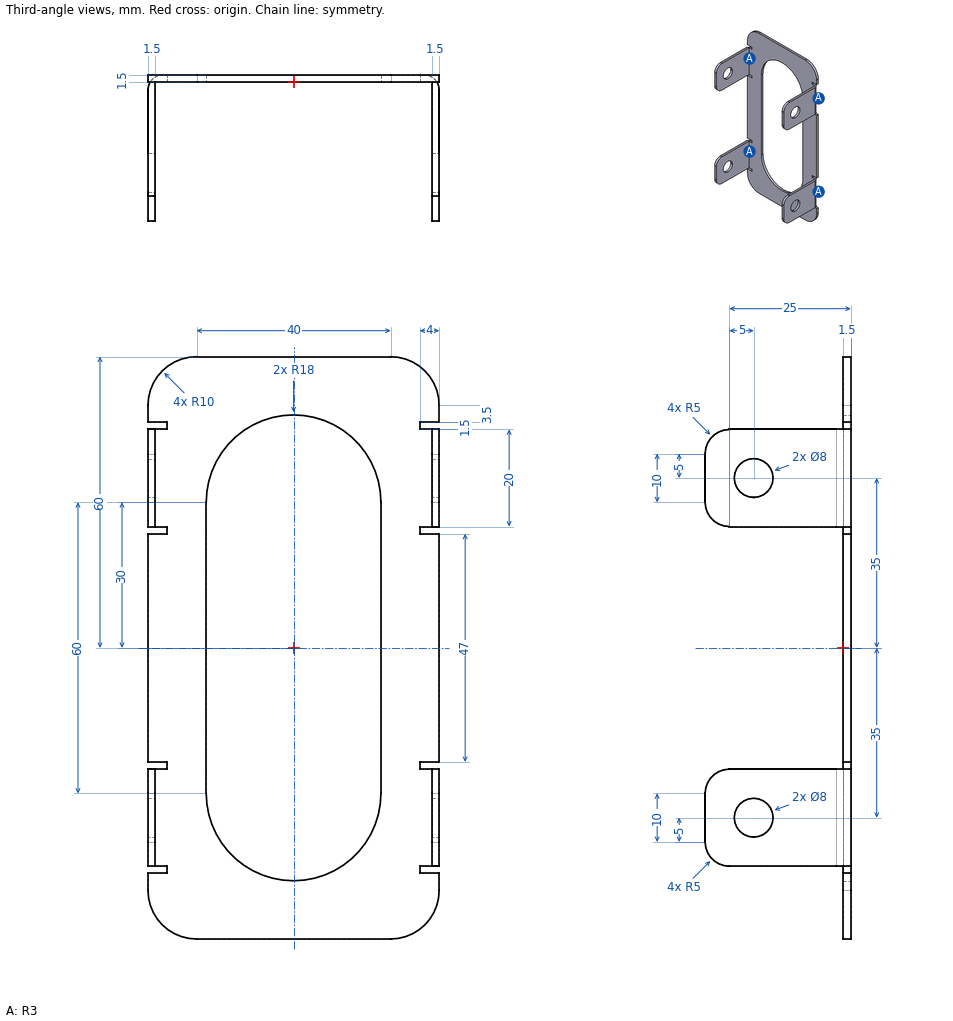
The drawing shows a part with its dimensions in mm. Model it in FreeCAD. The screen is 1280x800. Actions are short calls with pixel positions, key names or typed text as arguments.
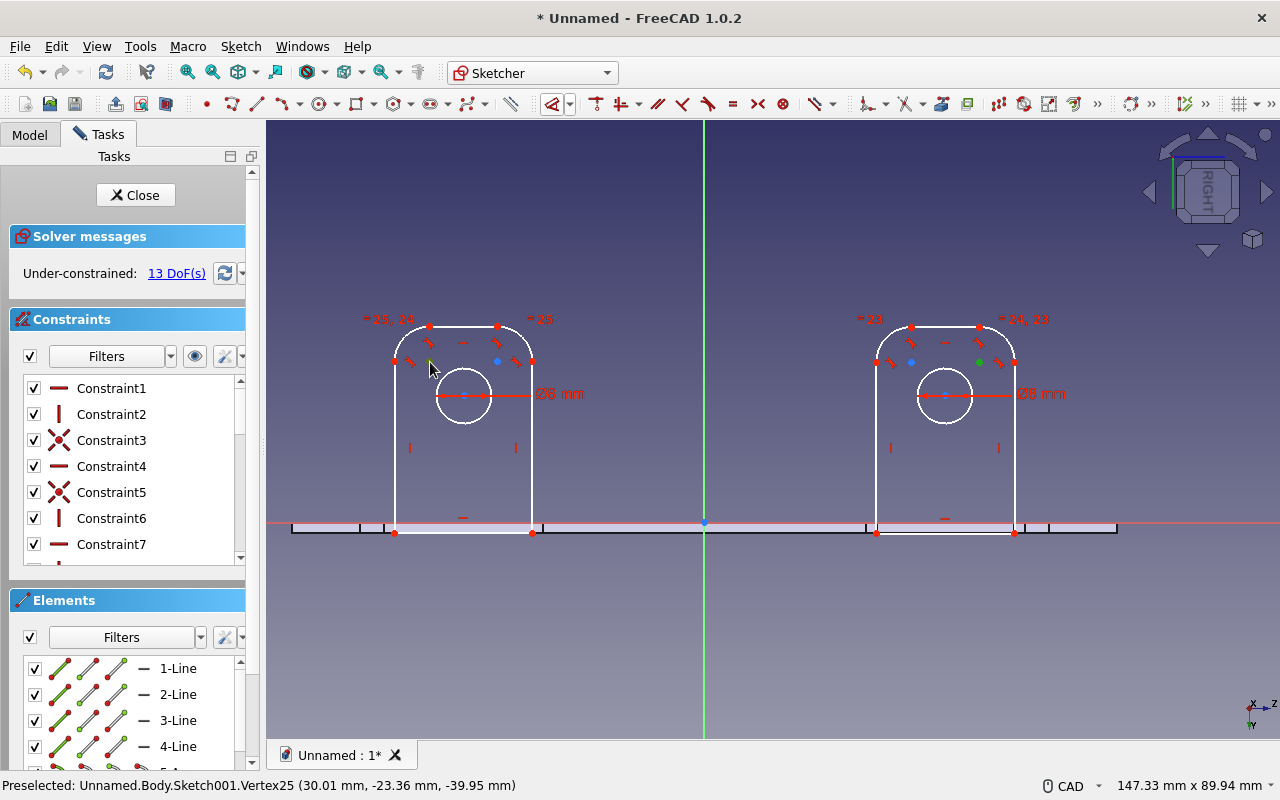
click(704, 671)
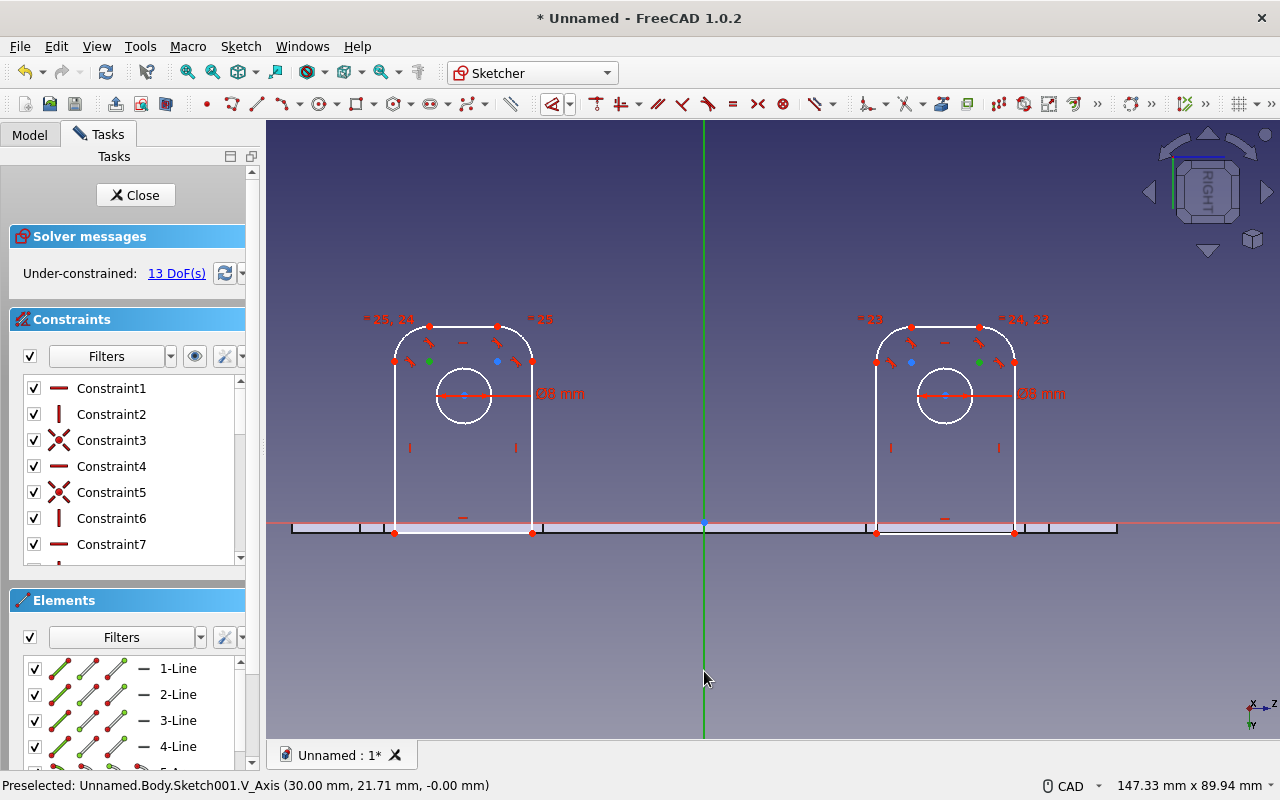
click(758, 104)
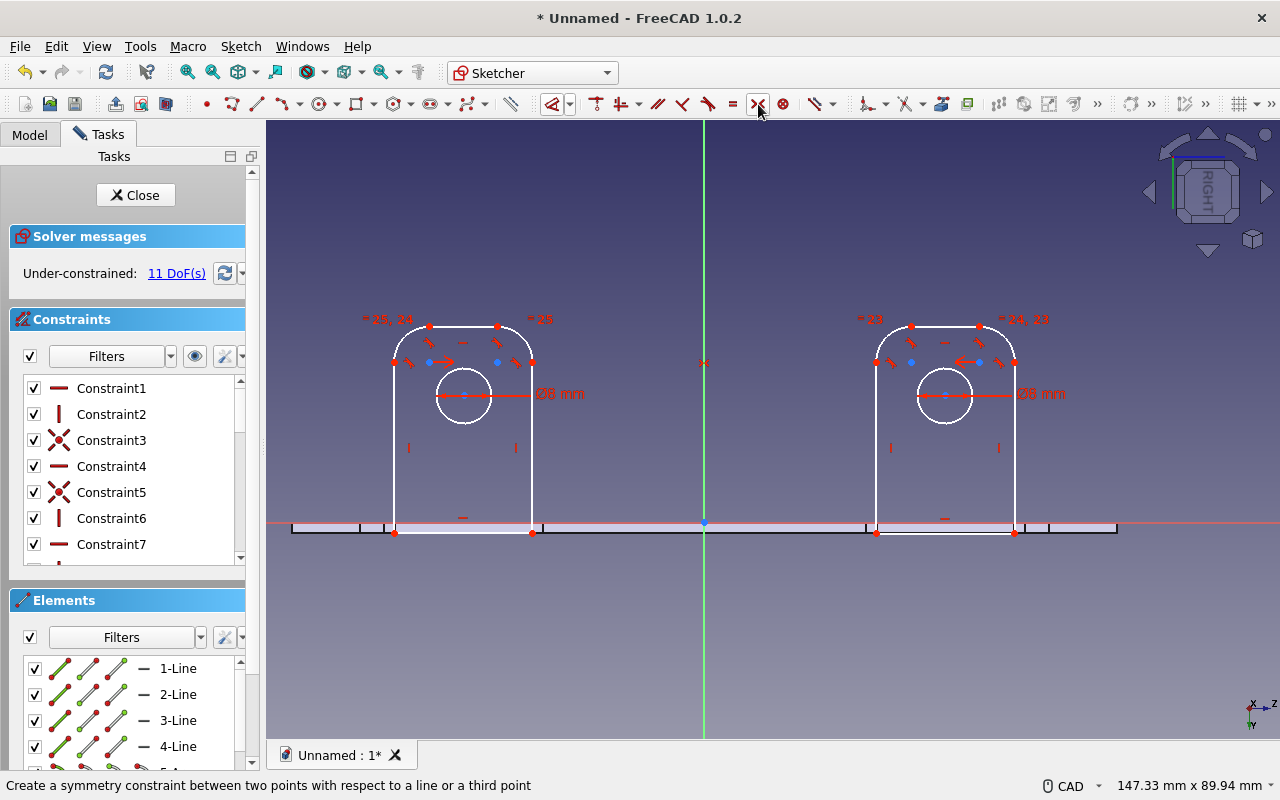
click(945, 396)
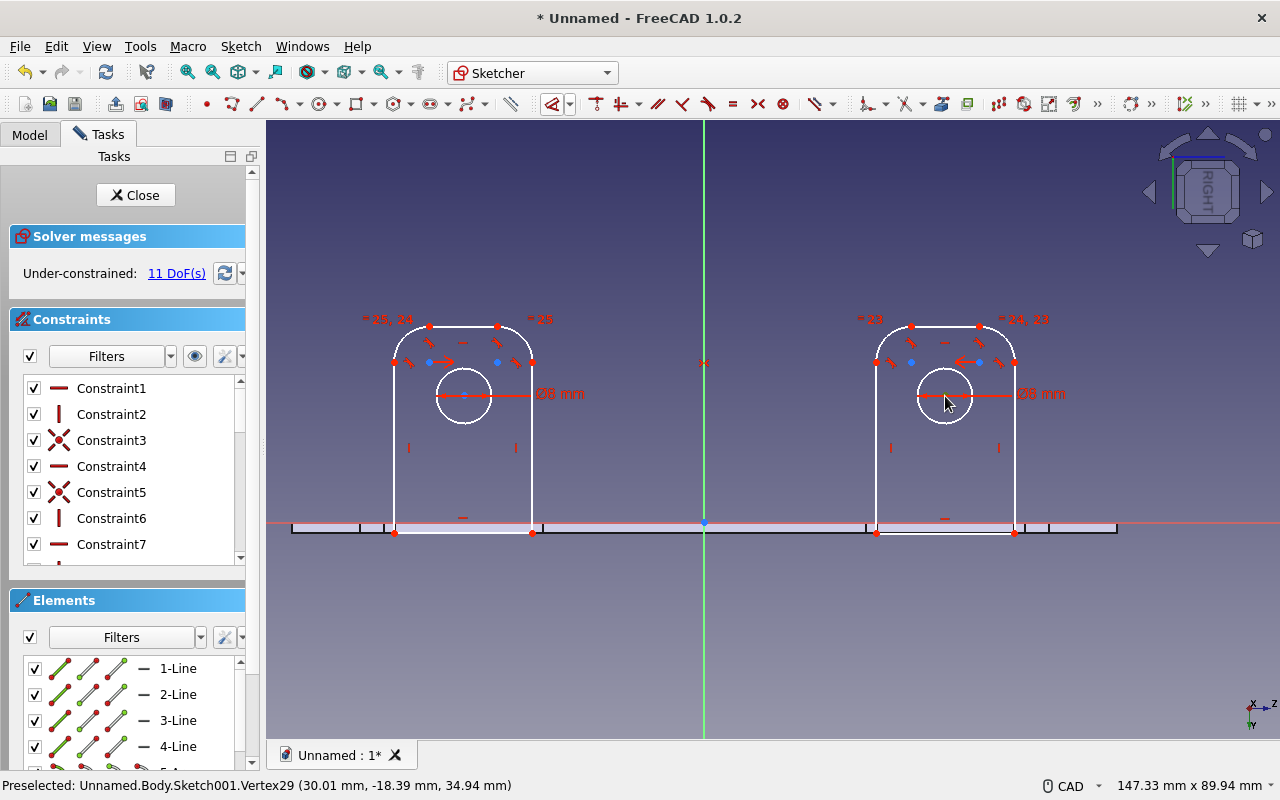
click(464, 396)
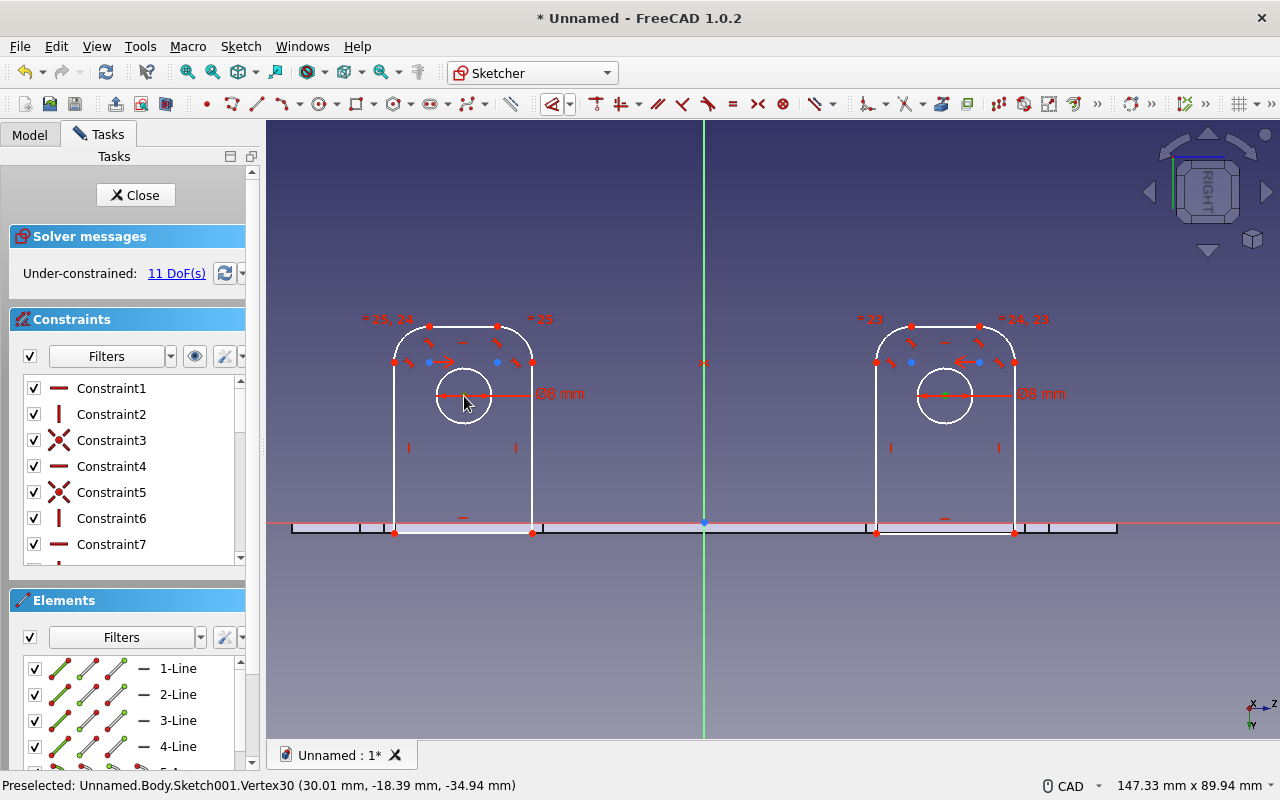
click(704, 671)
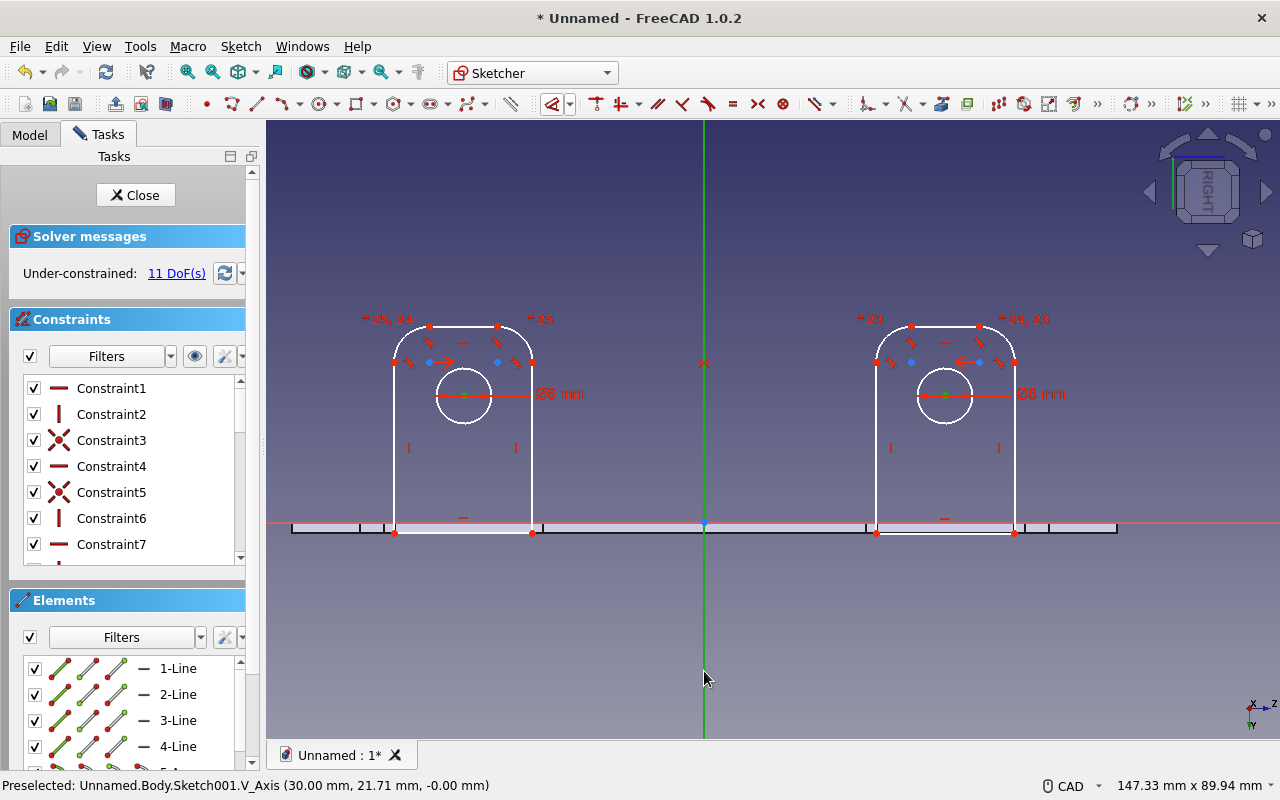
click(758, 104)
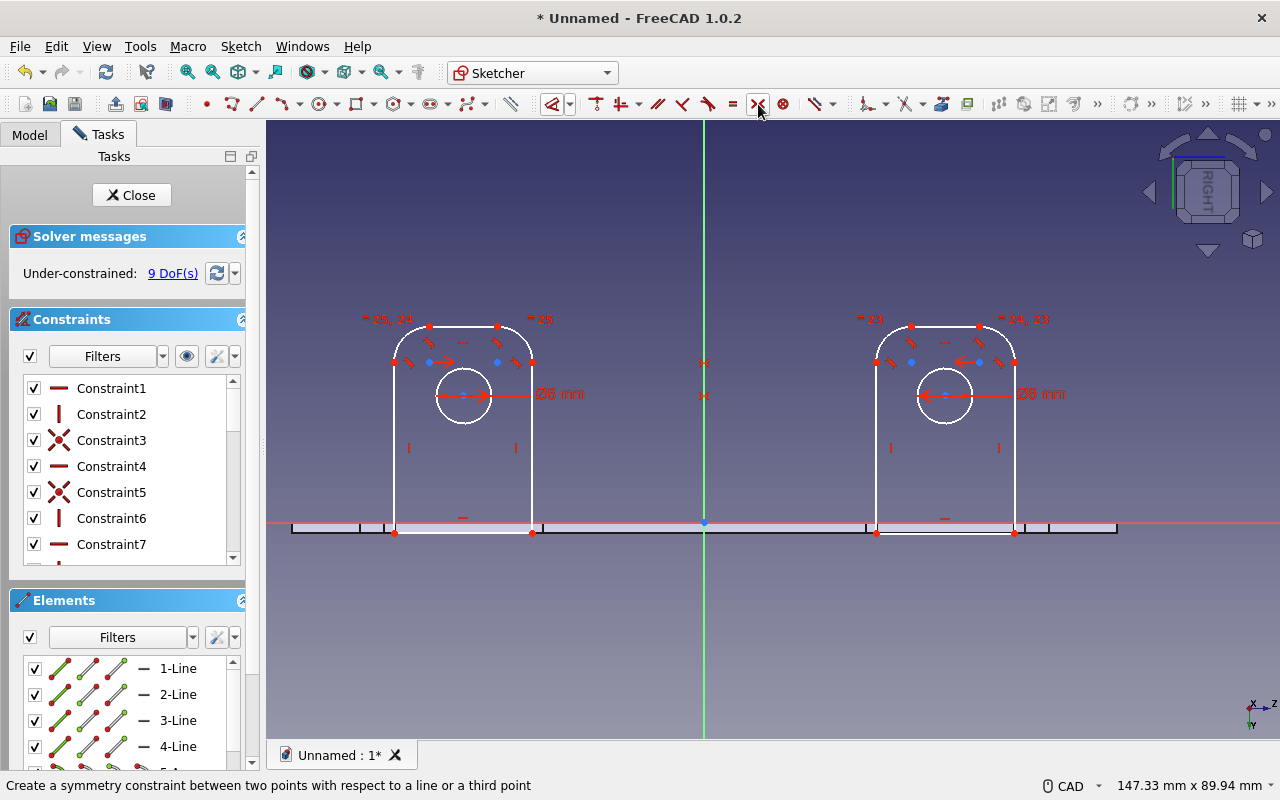
click(876, 534)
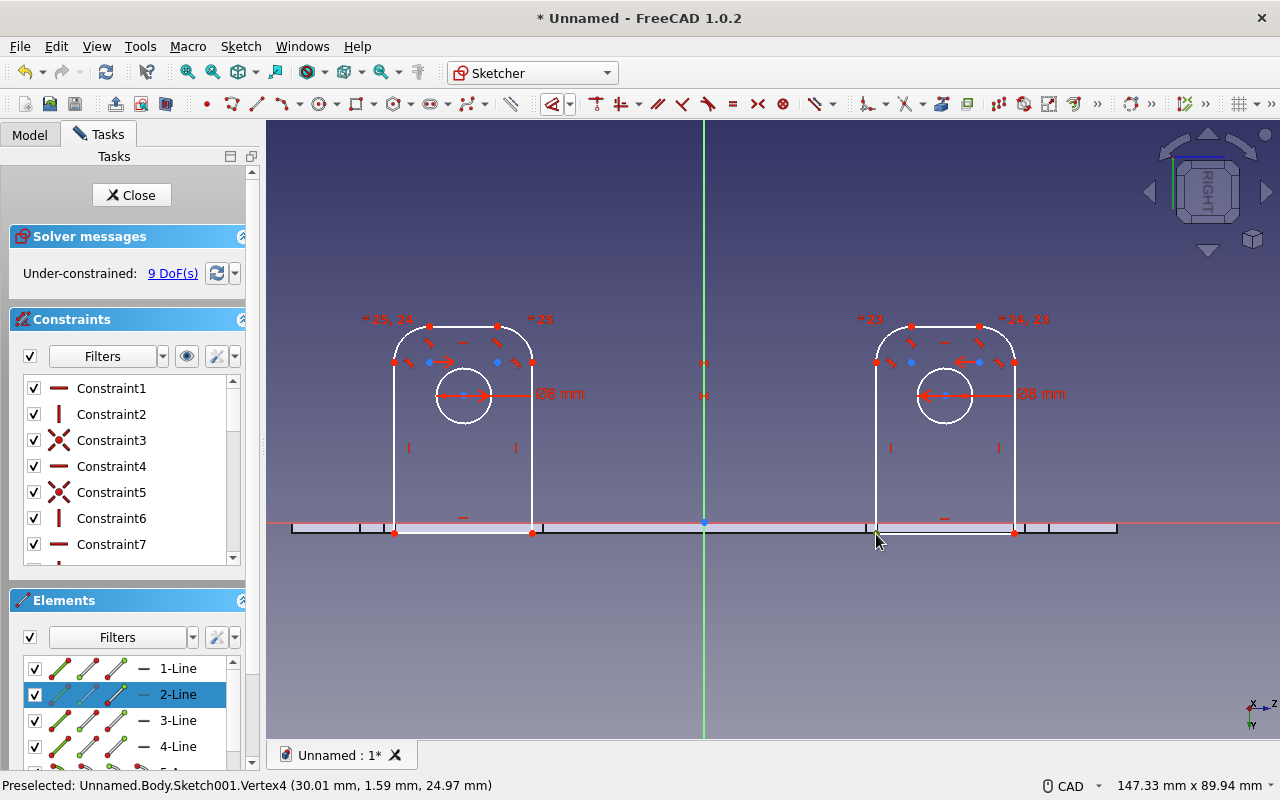
click(532, 533)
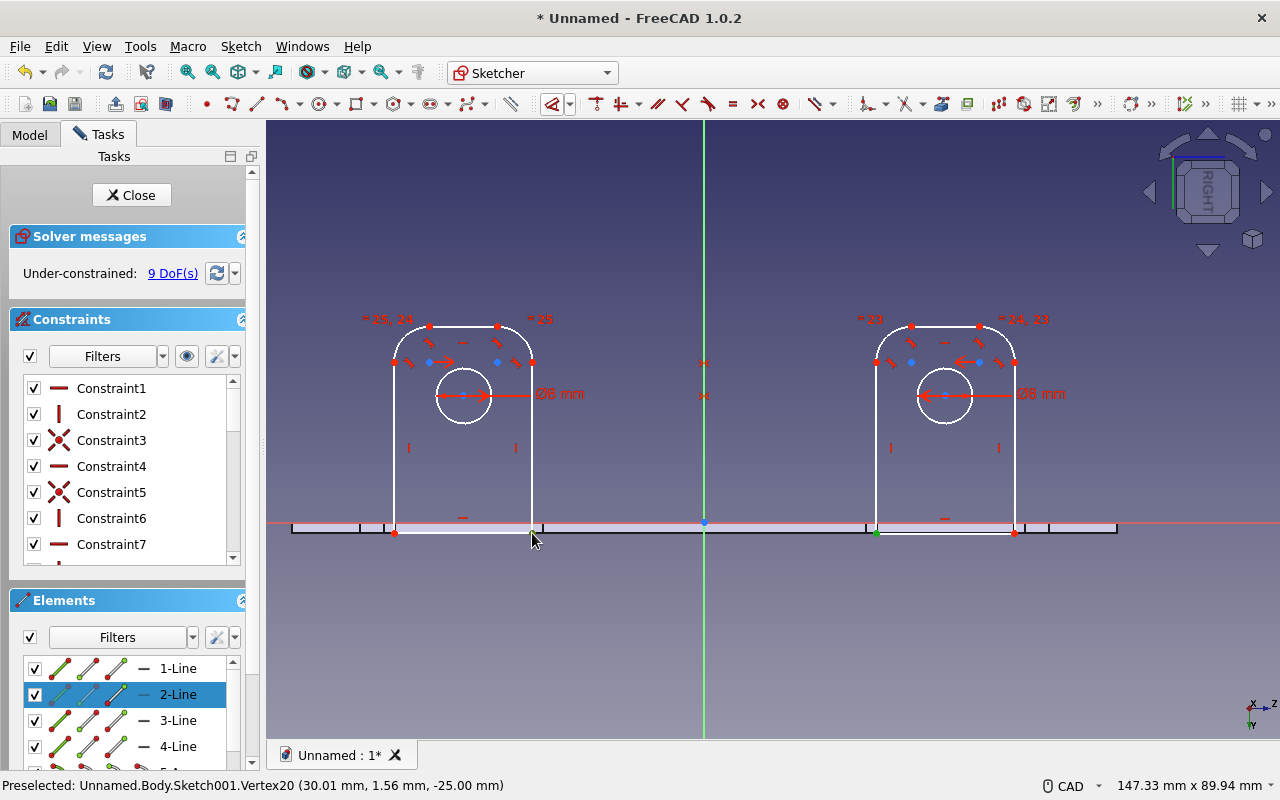
click(704, 671)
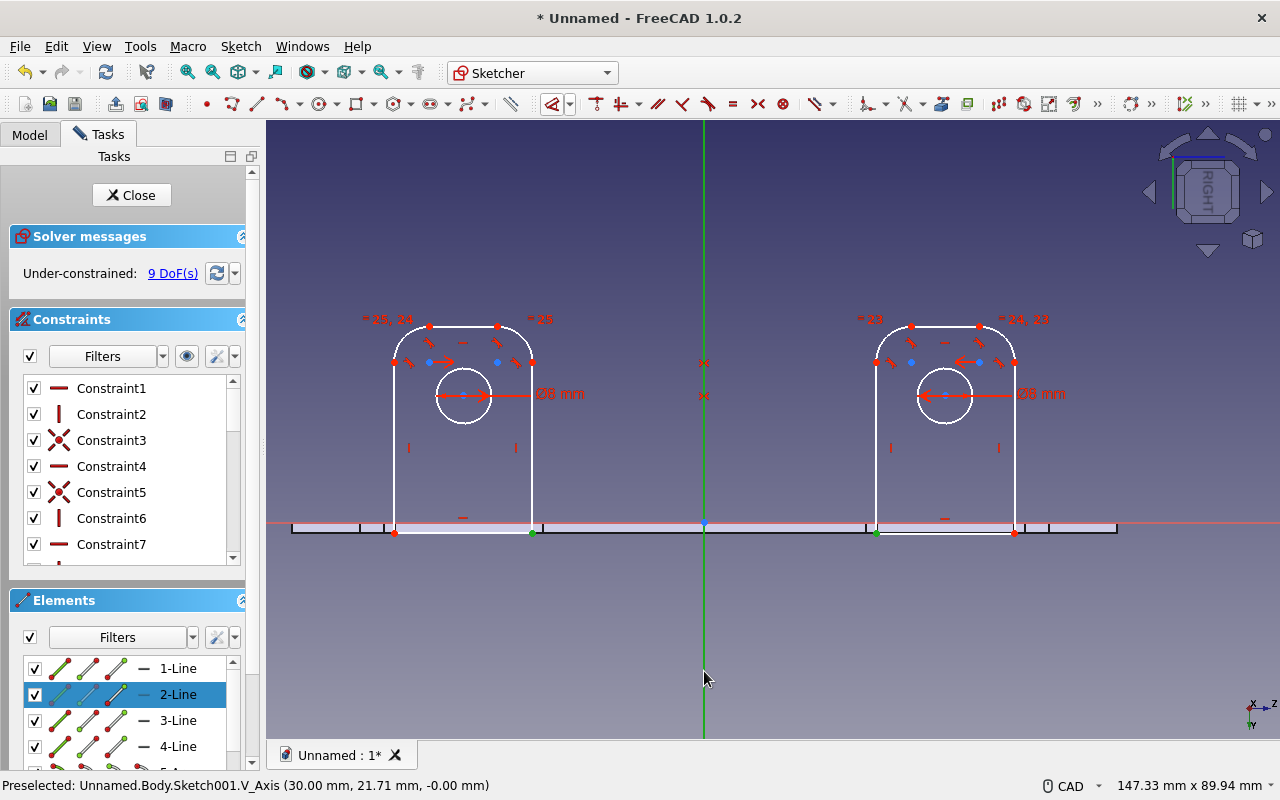
click(758, 104)